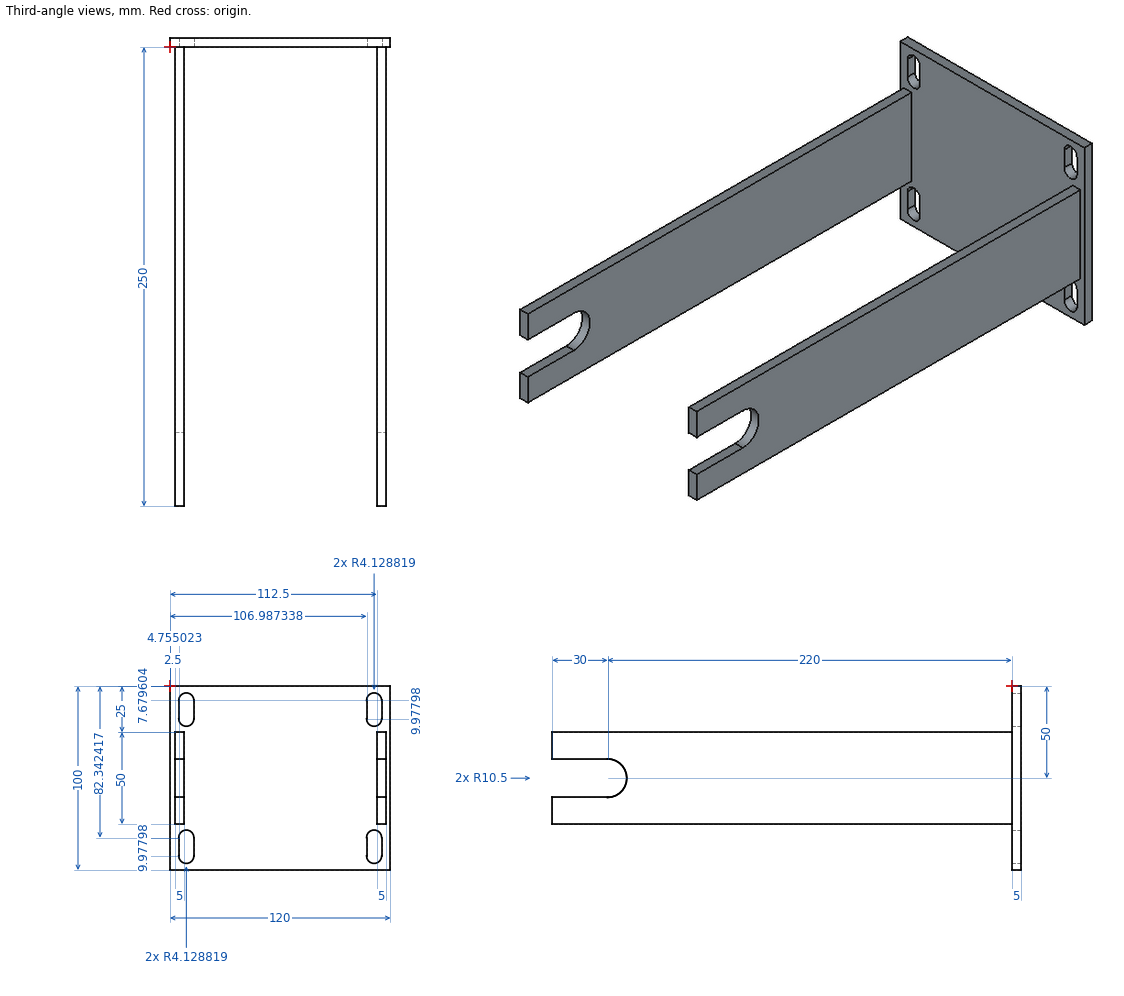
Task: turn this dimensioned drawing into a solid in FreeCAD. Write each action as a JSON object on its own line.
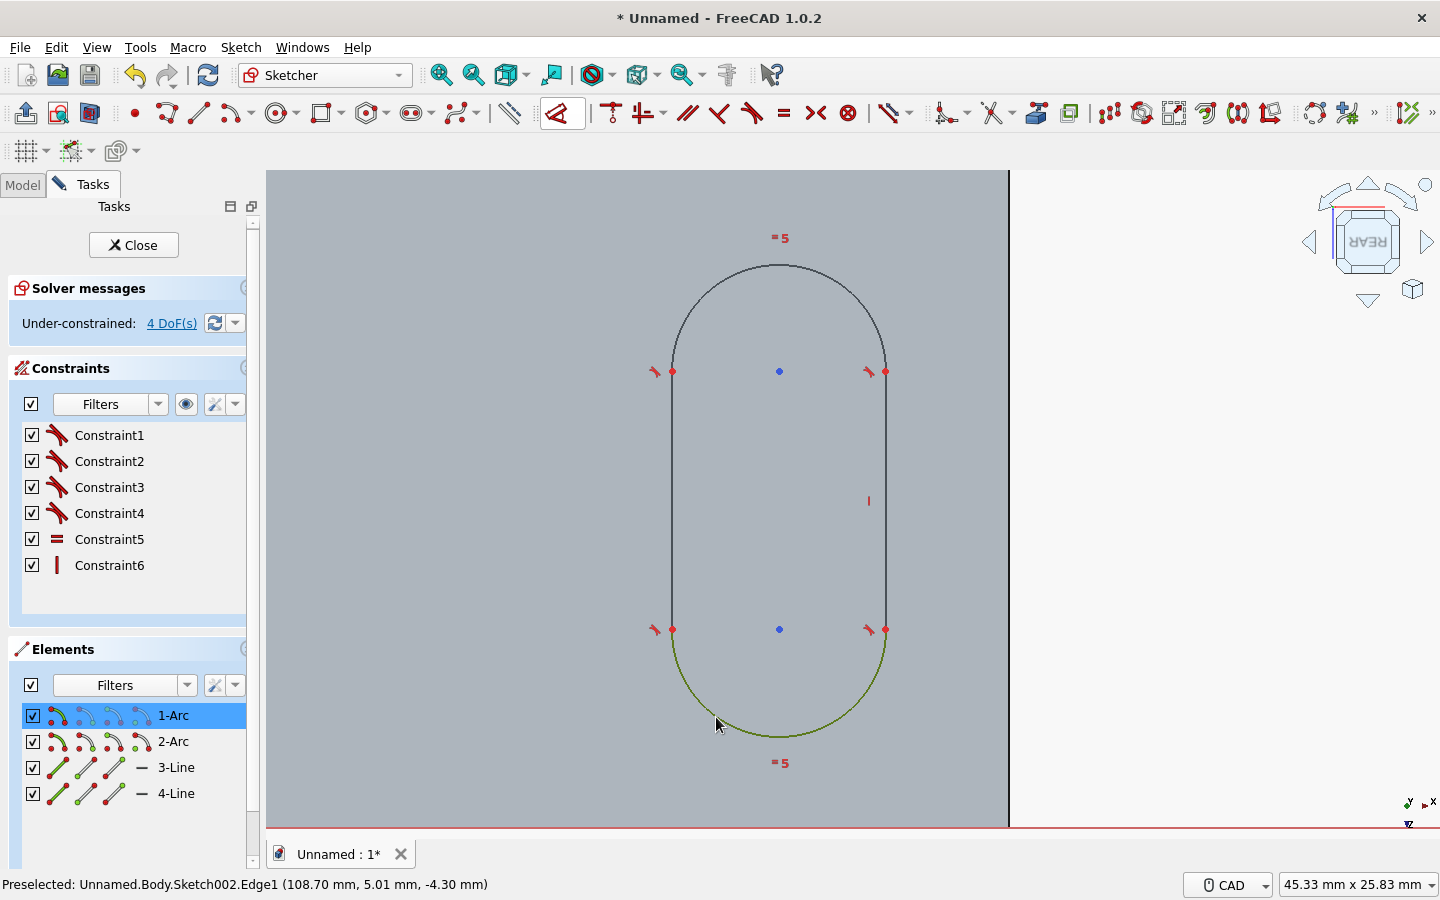
{"action": "left_click", "coordinate": [580, 114]}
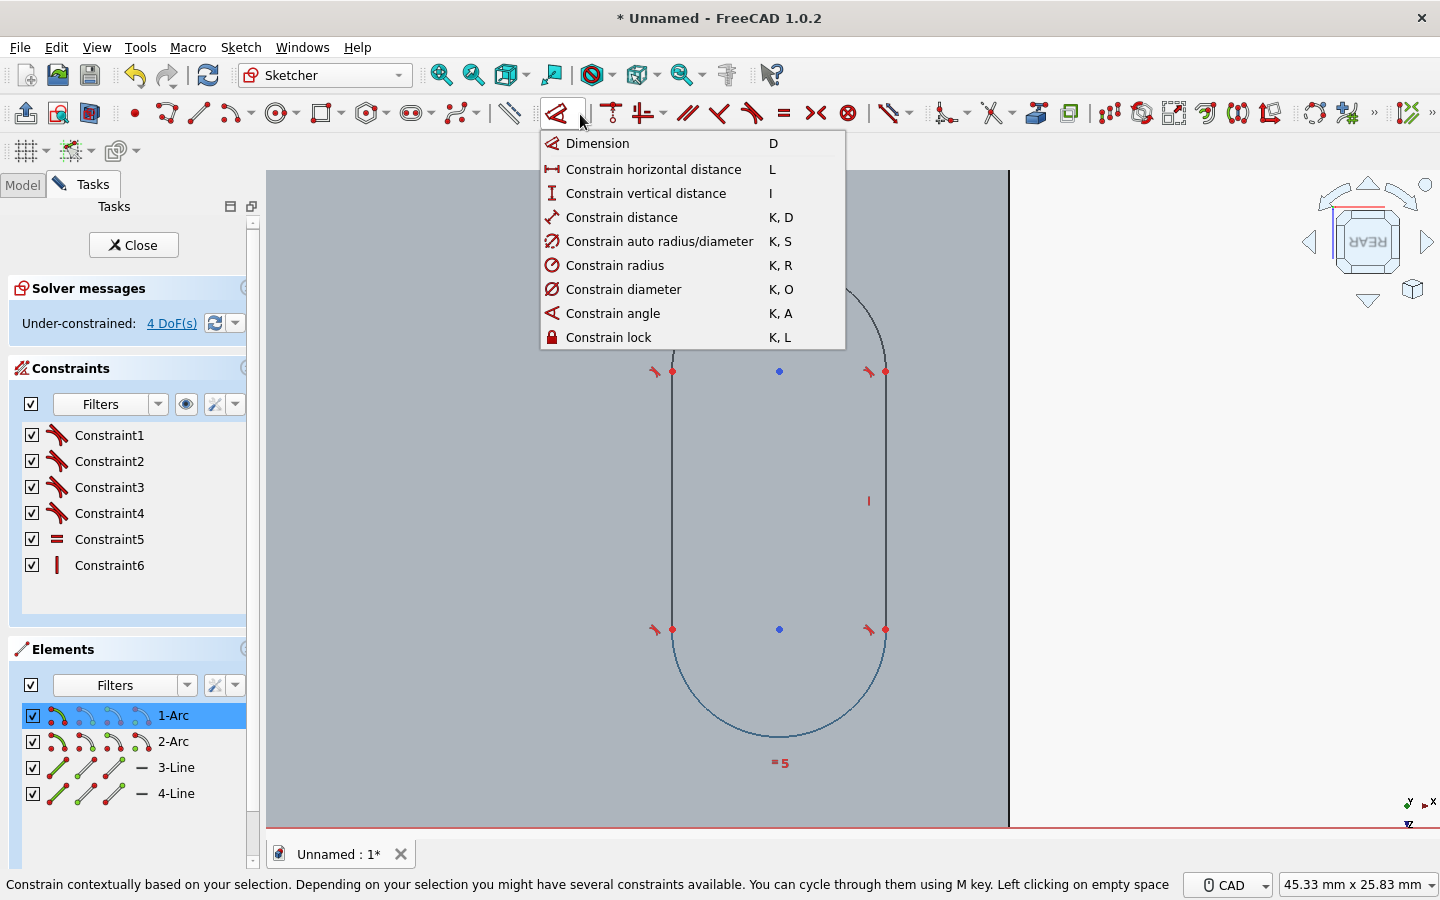
{"action": "left_click", "coordinate": [693, 265]}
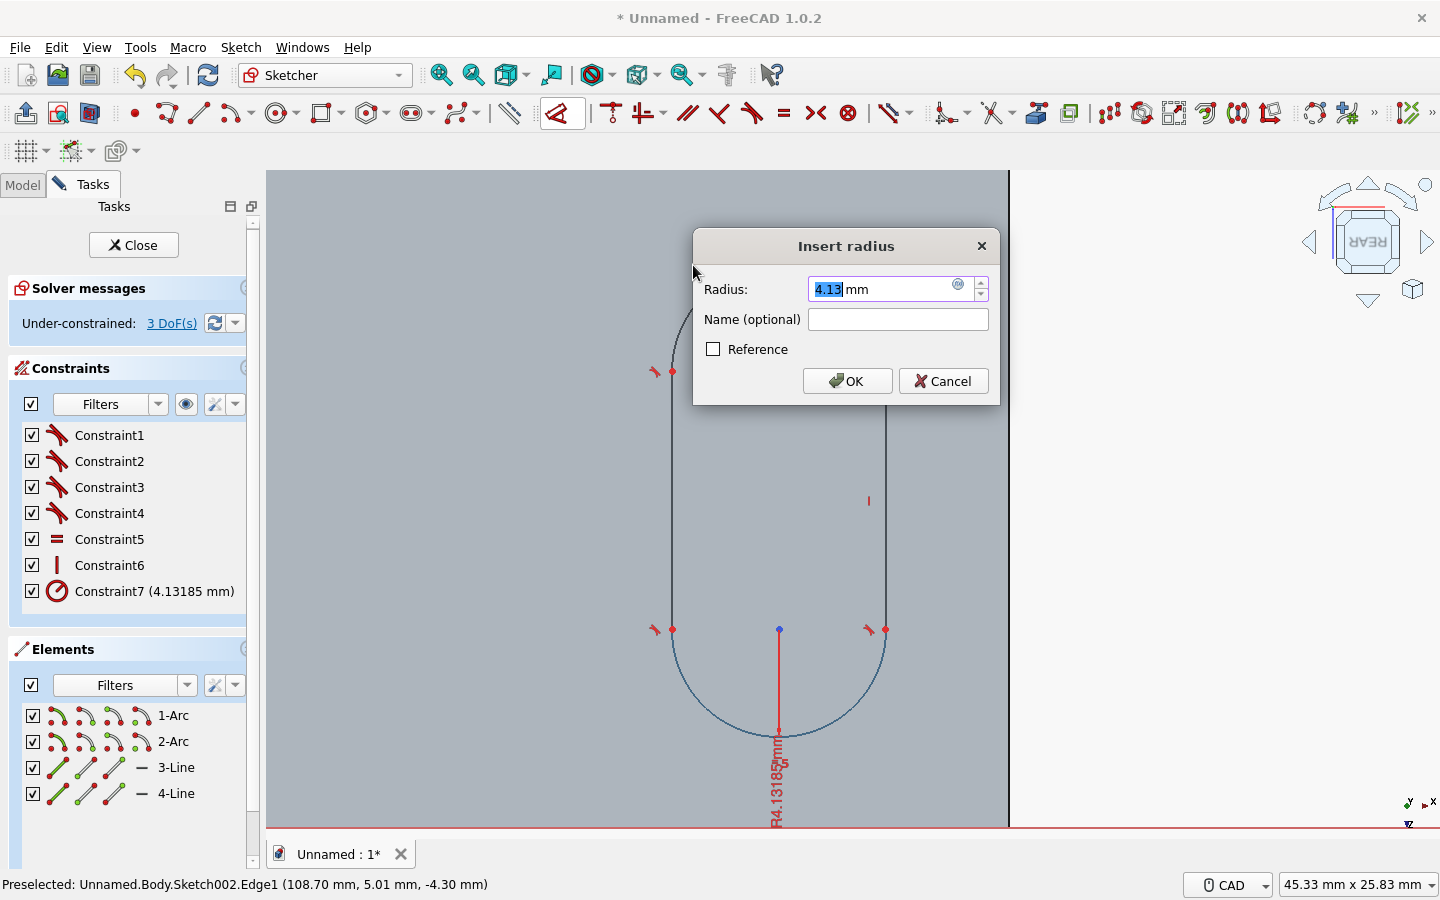
{"action": "type", "text": "4.128819"}
{"action": "key", "text": "Return"}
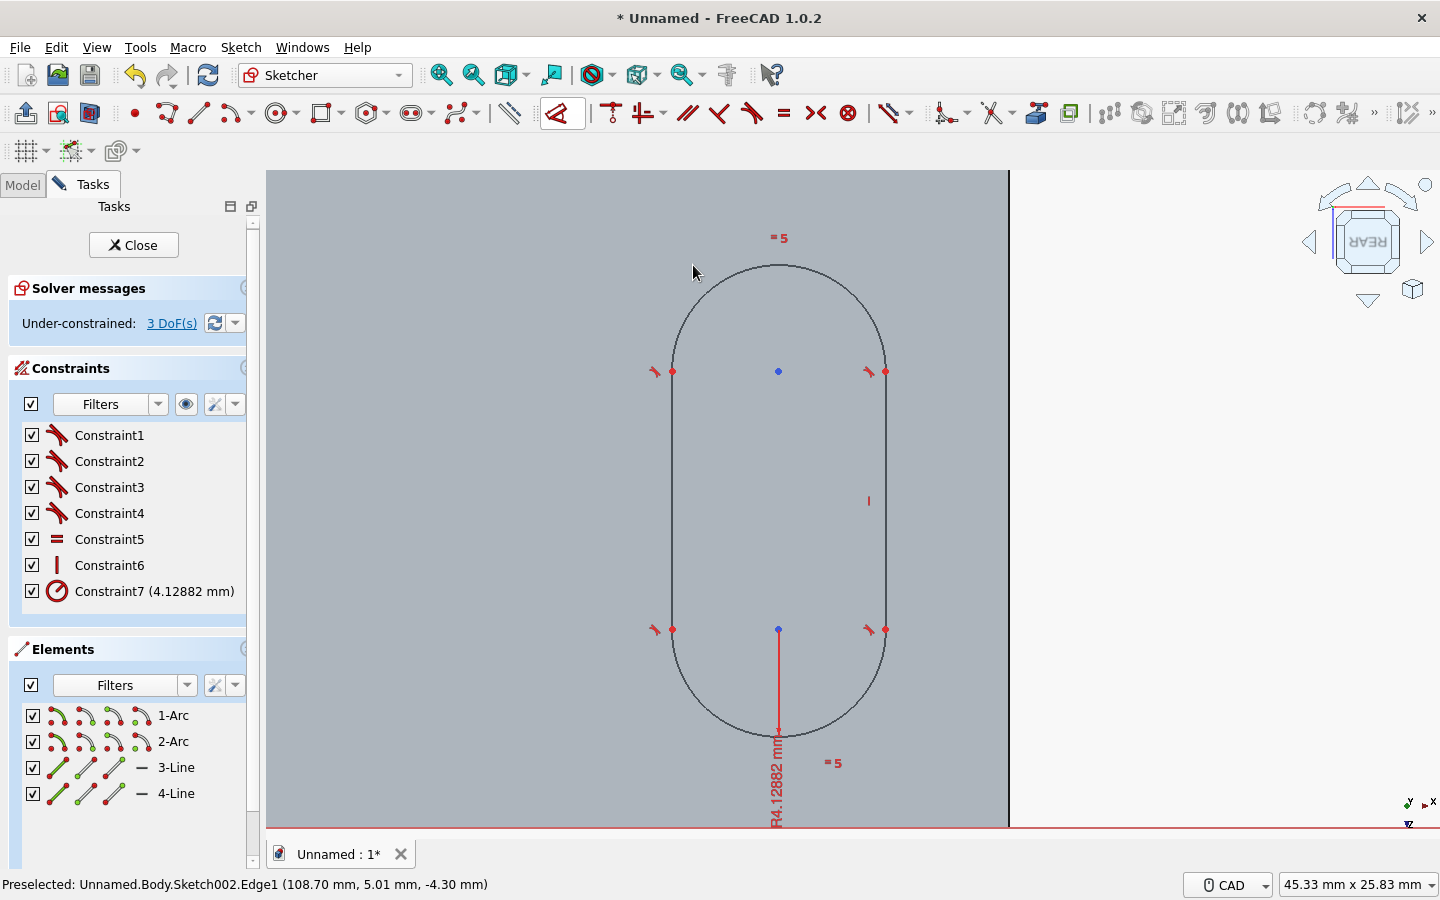
{"action": "left_click", "coordinate": [672, 553]}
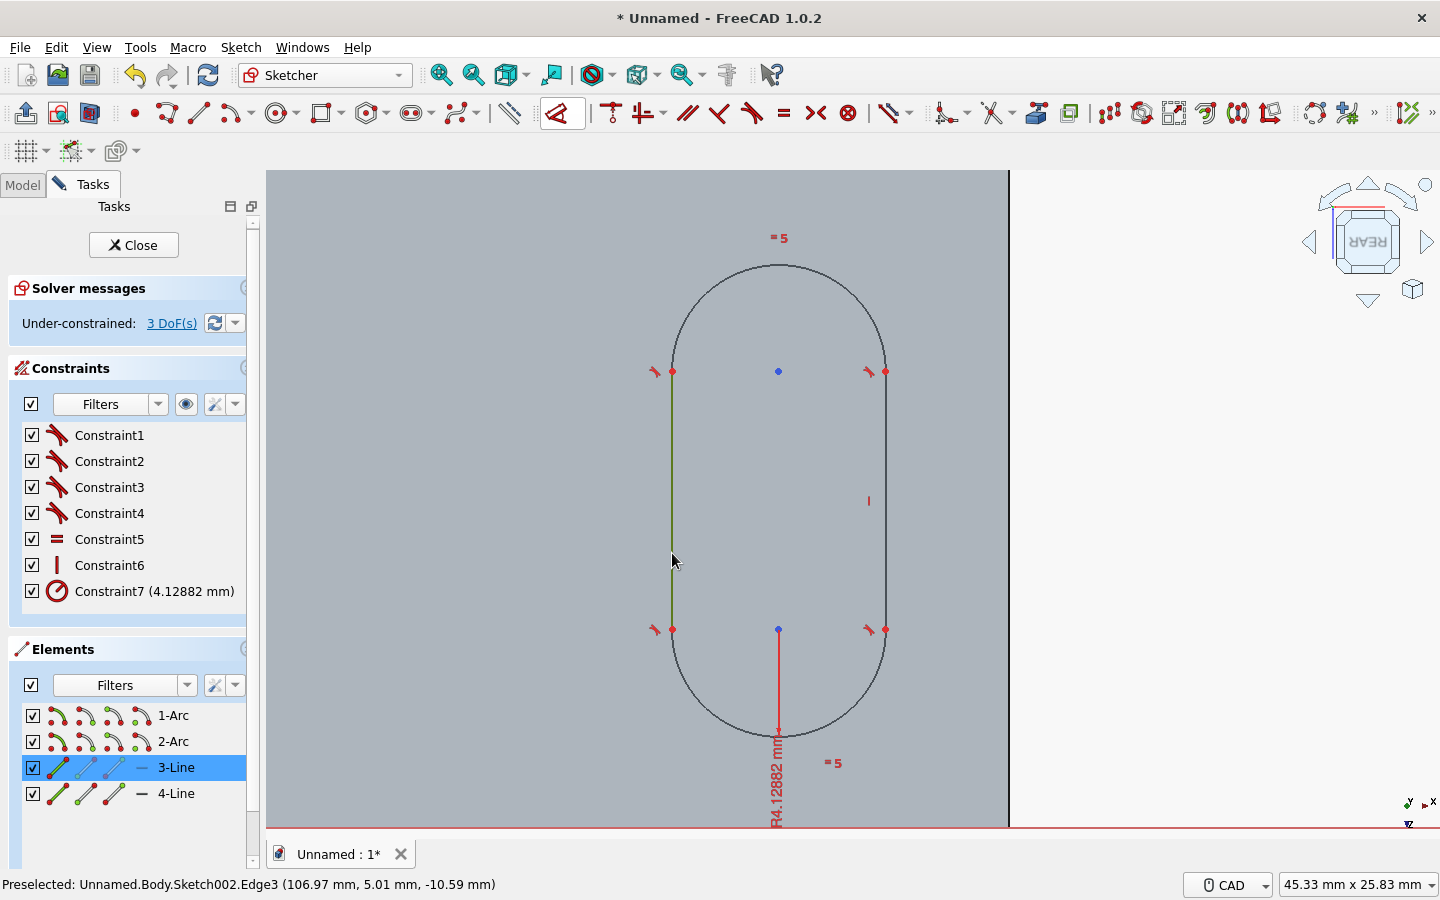
{"action": "left_click", "coordinate": [580, 114]}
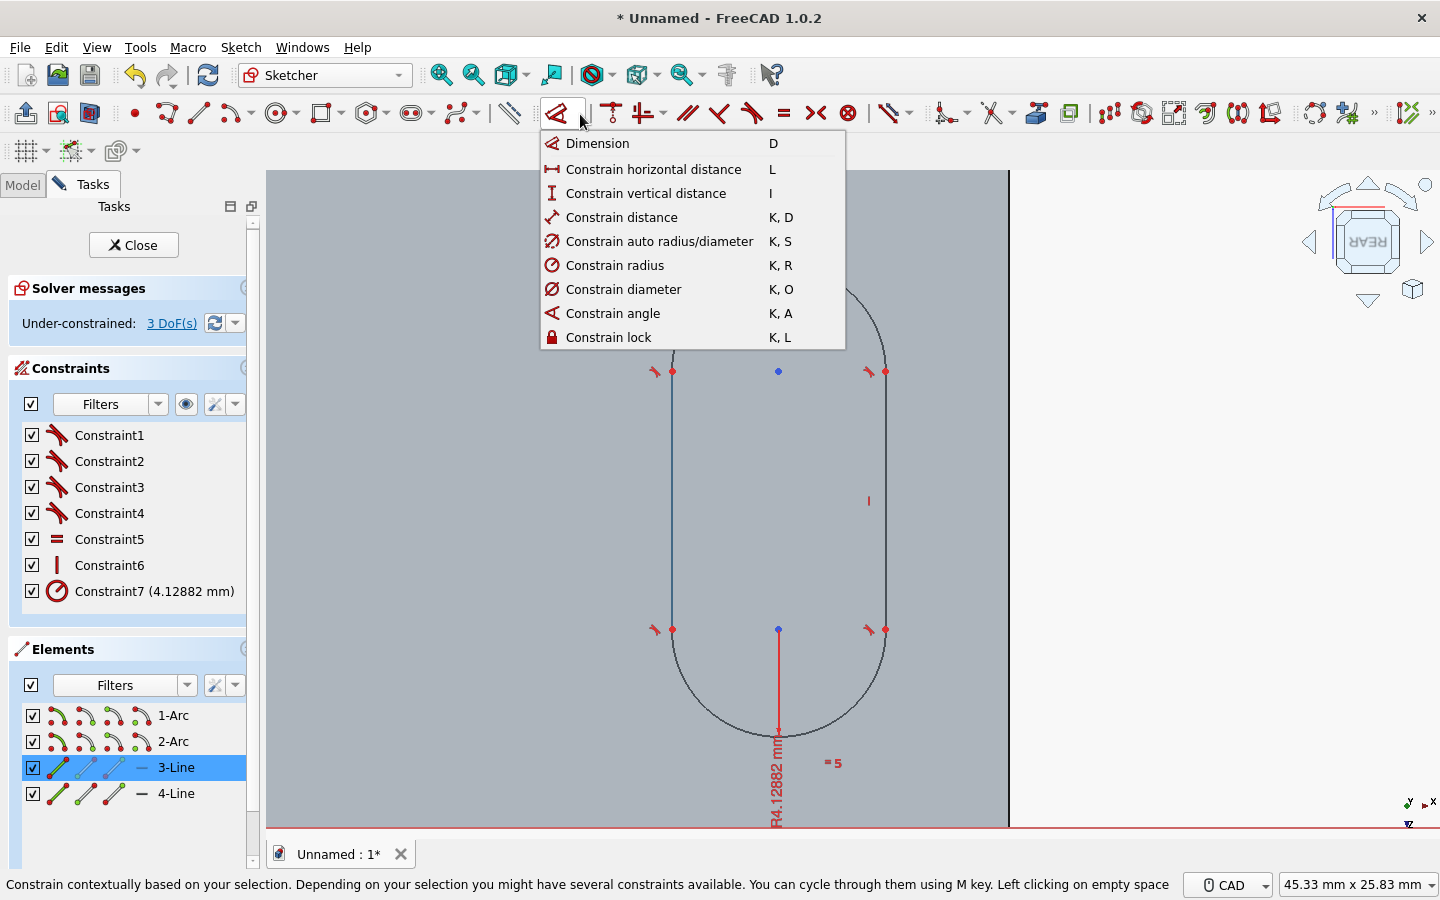
{"action": "left_click", "coordinate": [693, 193]}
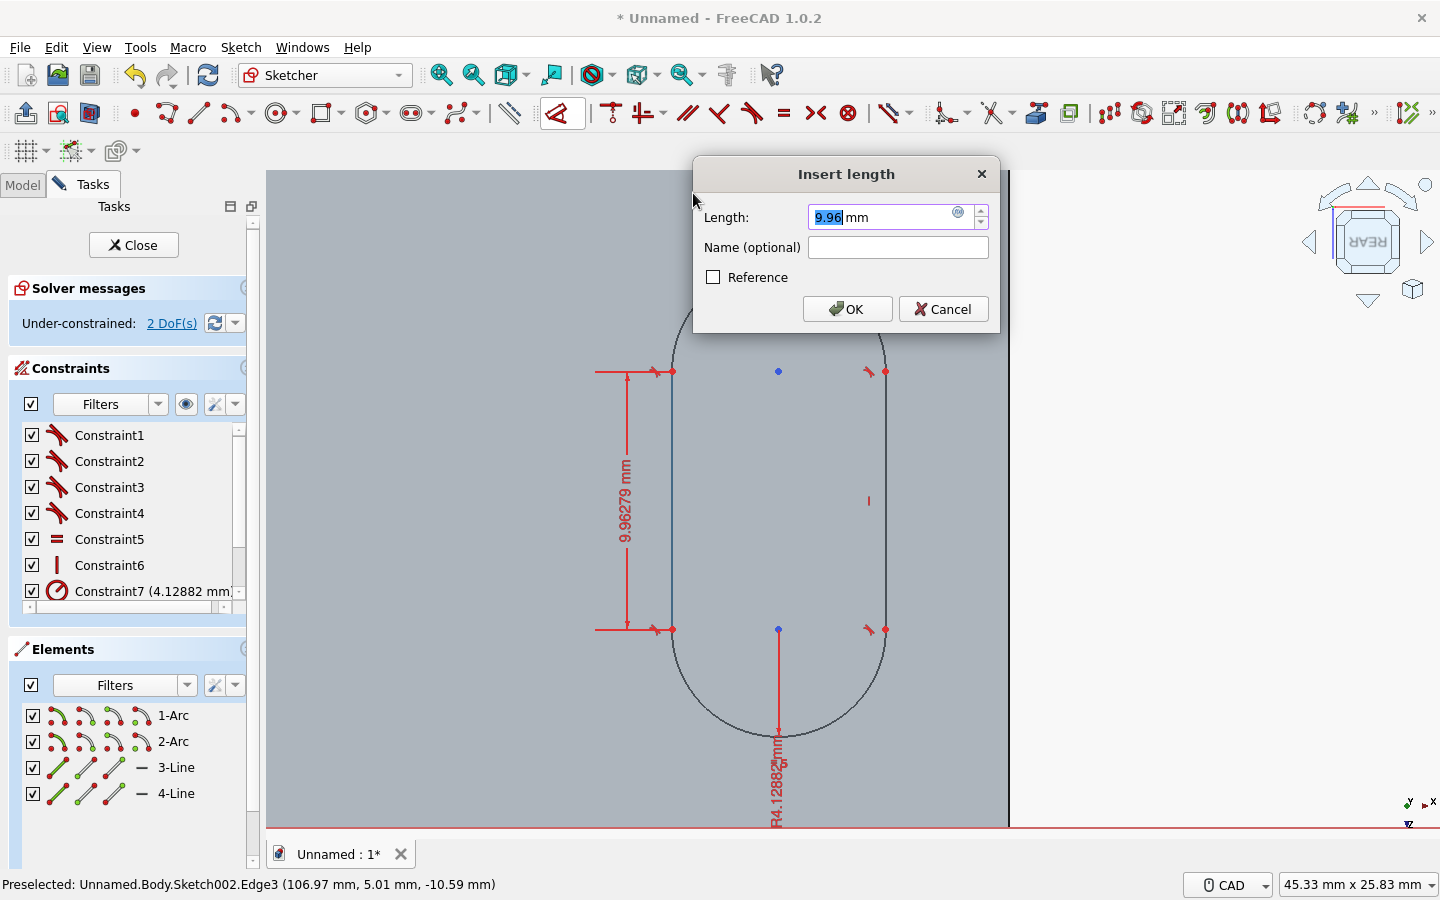
{"action": "type", "text": "9.97798"}
{"action": "key", "text": "Return"}